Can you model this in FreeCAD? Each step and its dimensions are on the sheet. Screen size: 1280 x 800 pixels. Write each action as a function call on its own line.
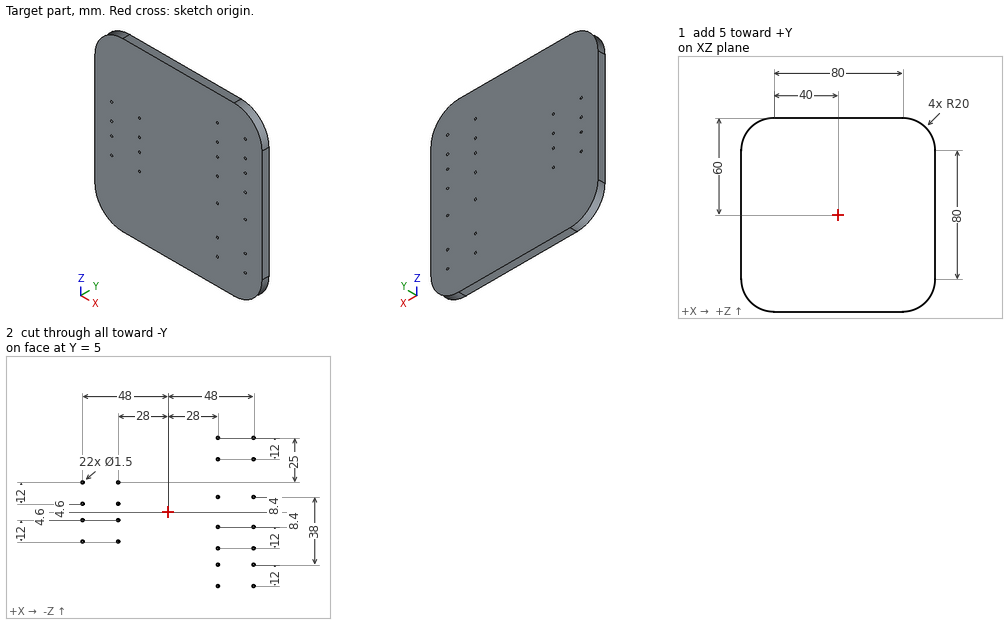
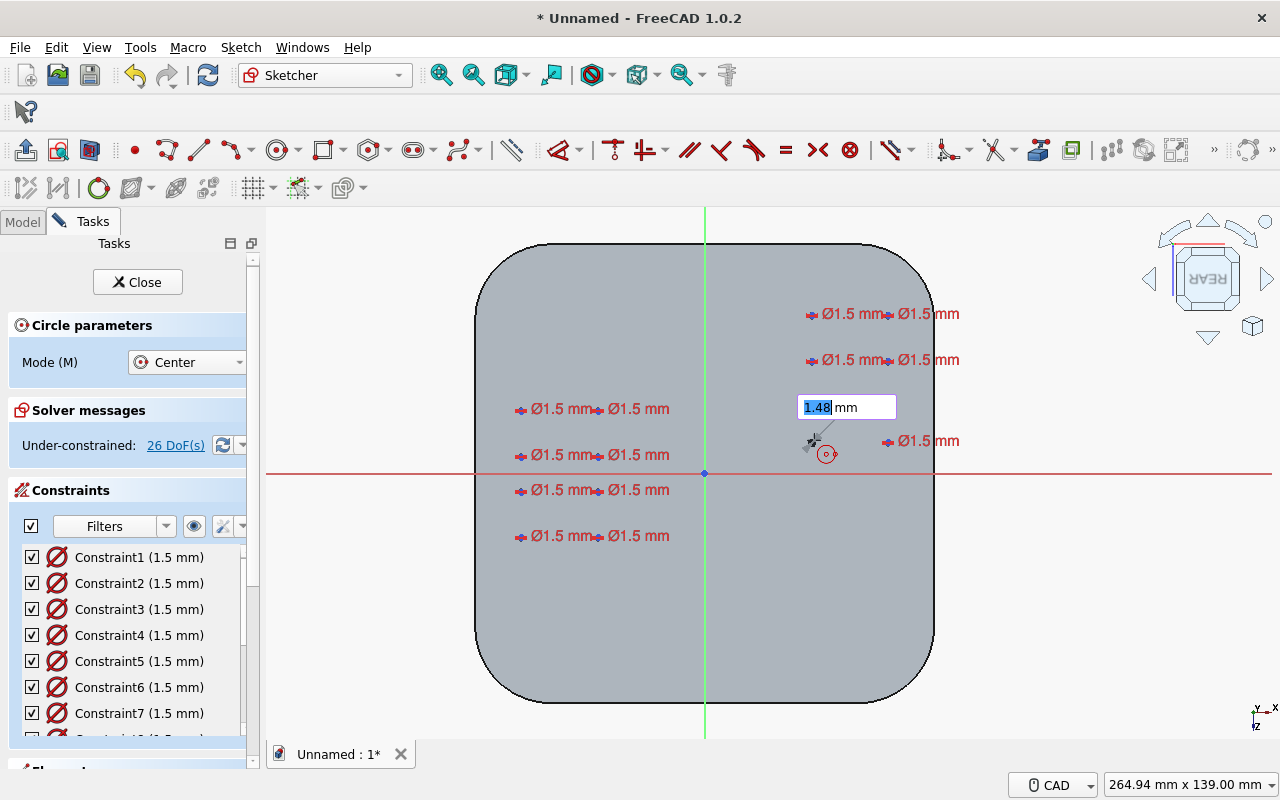
text(1.5)
key(Return)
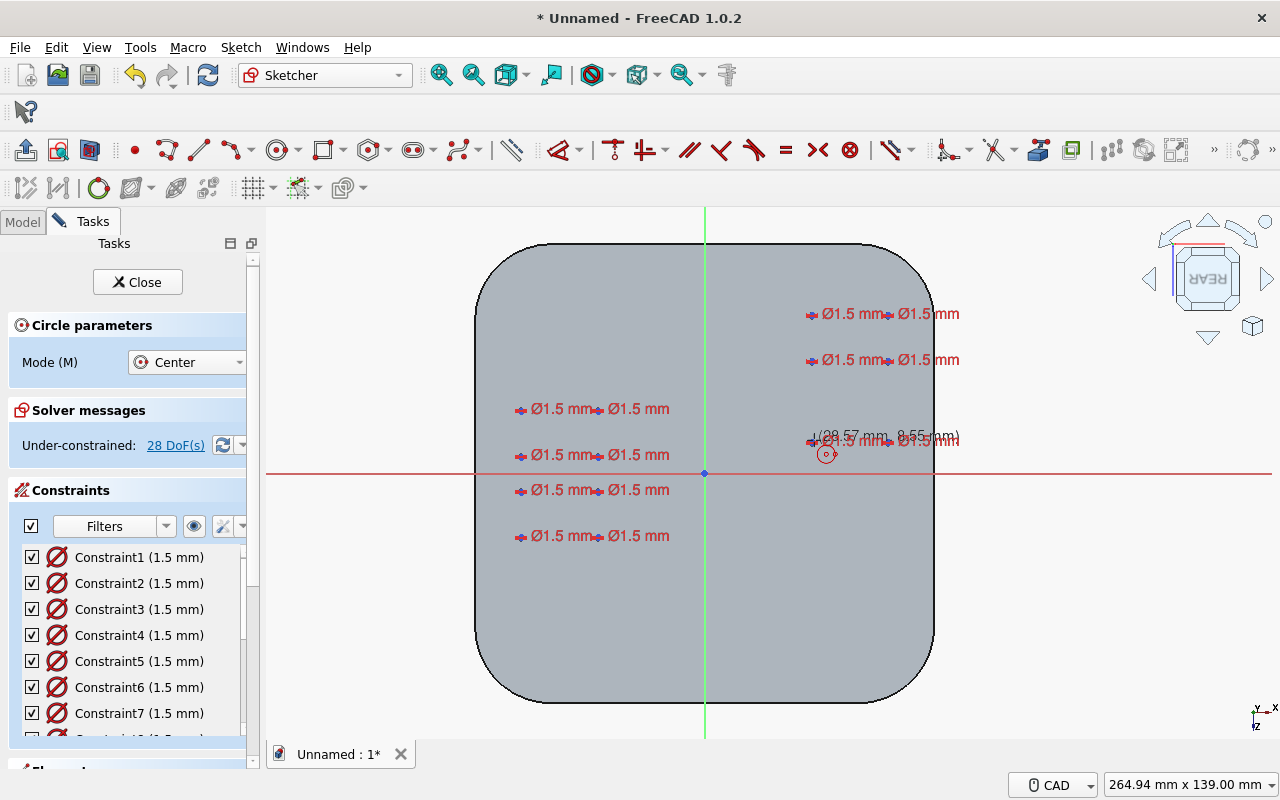
scroll(812, 506, up, 11)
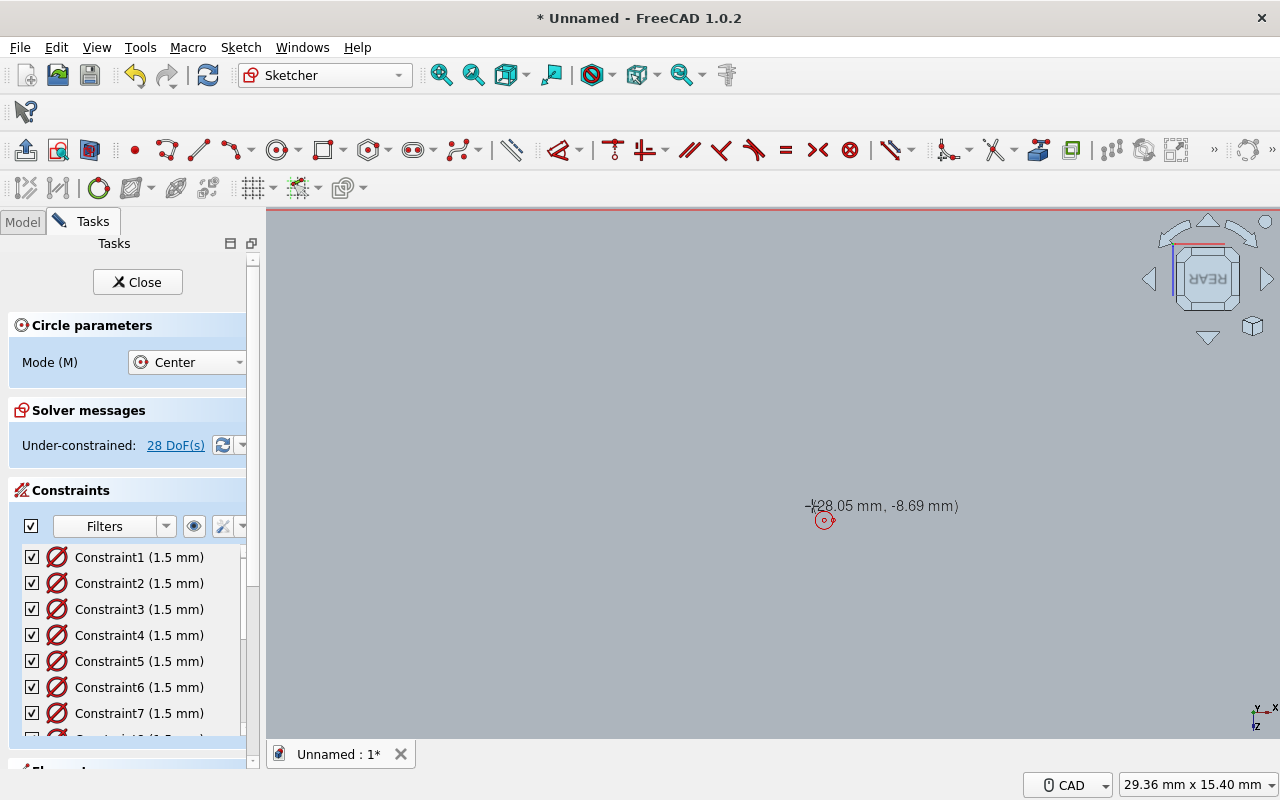
scroll(812, 506, down, 11)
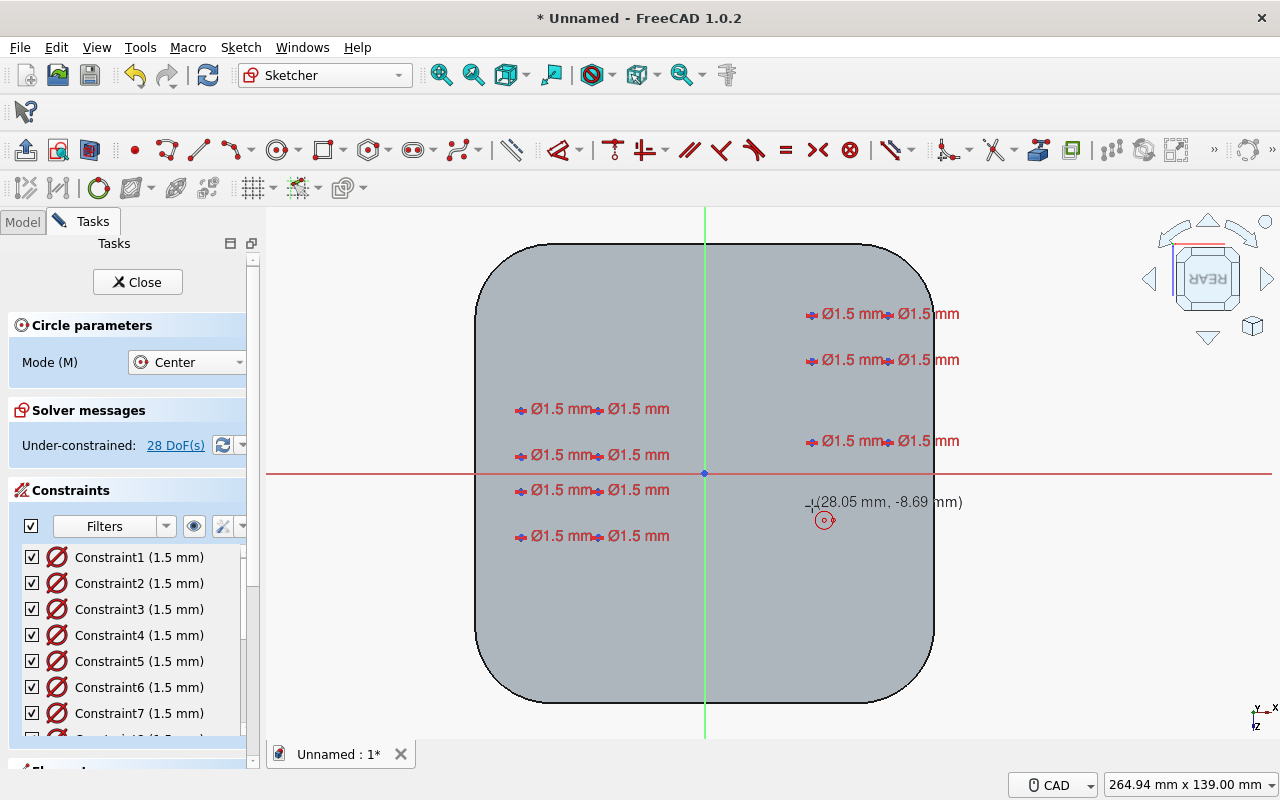
click(812, 506)
move(814, 504)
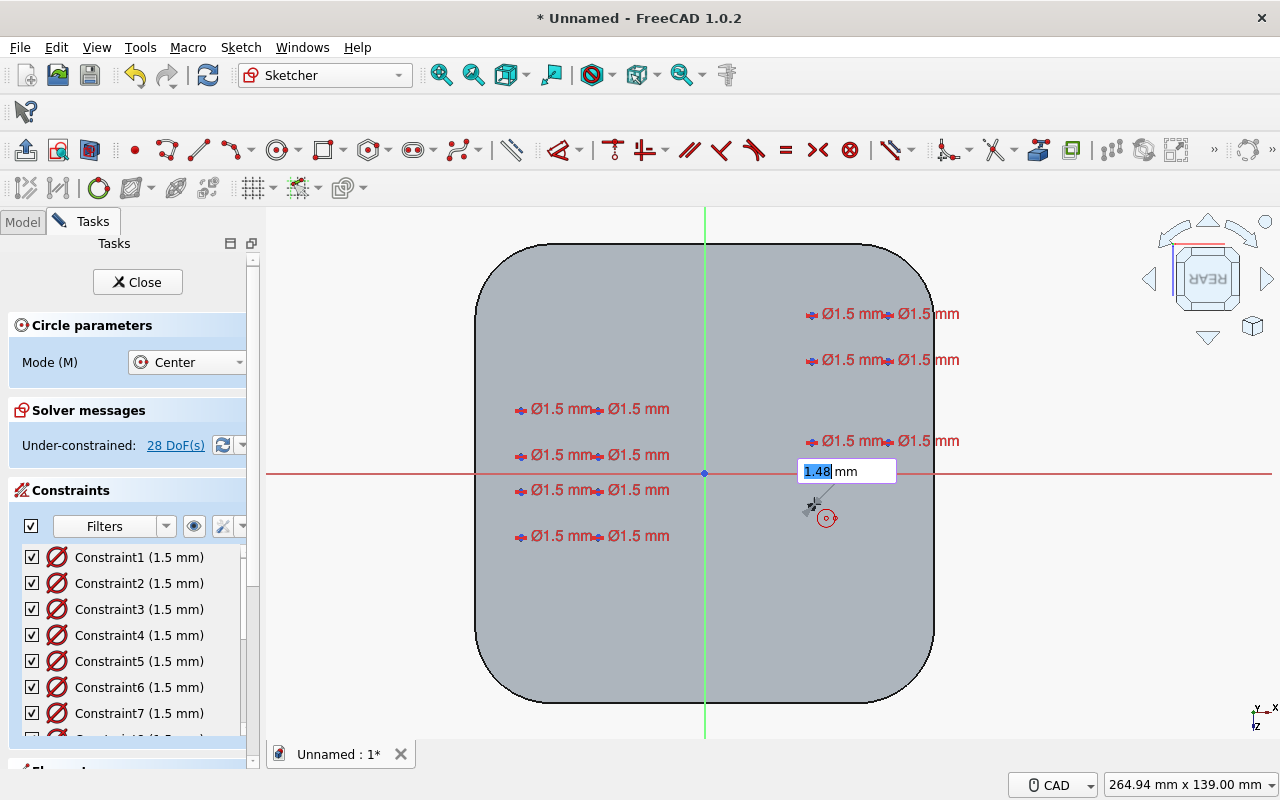
text(1.5)
key(Return)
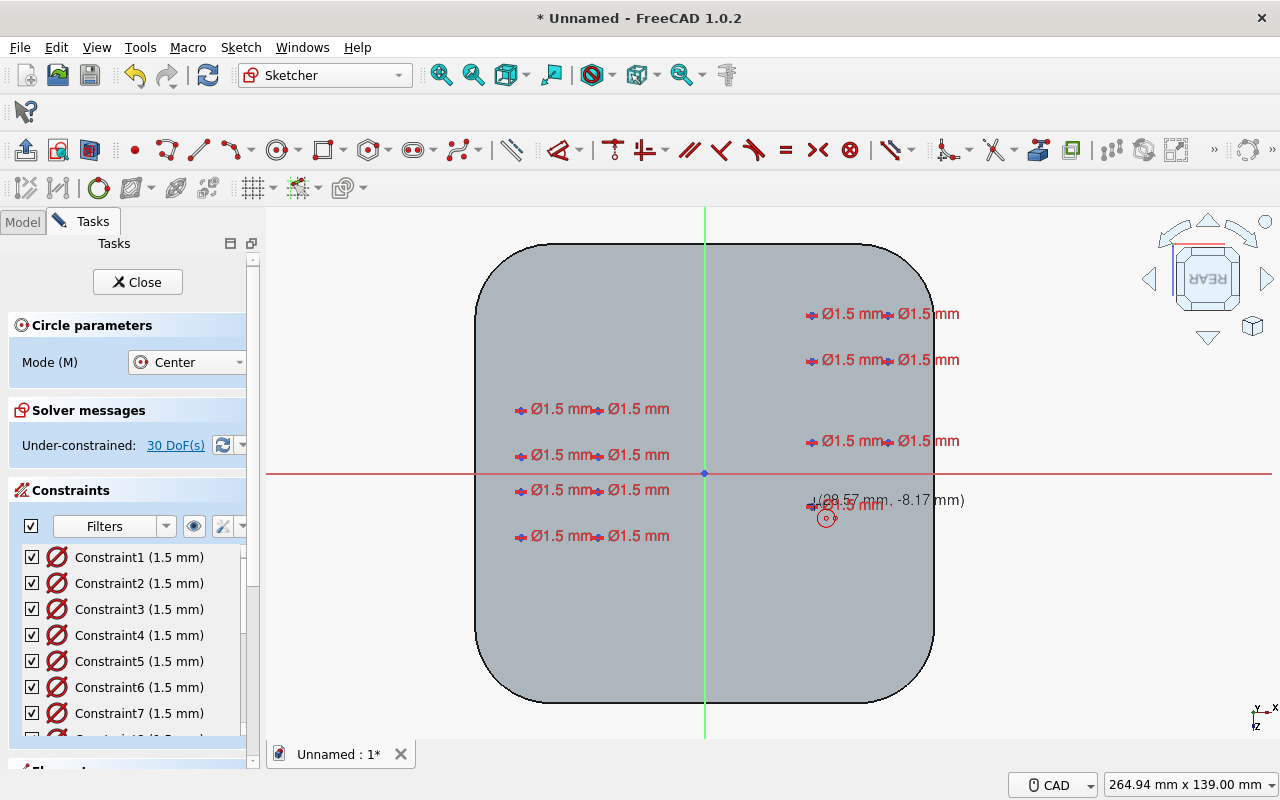
scroll(888, 506, up, 11)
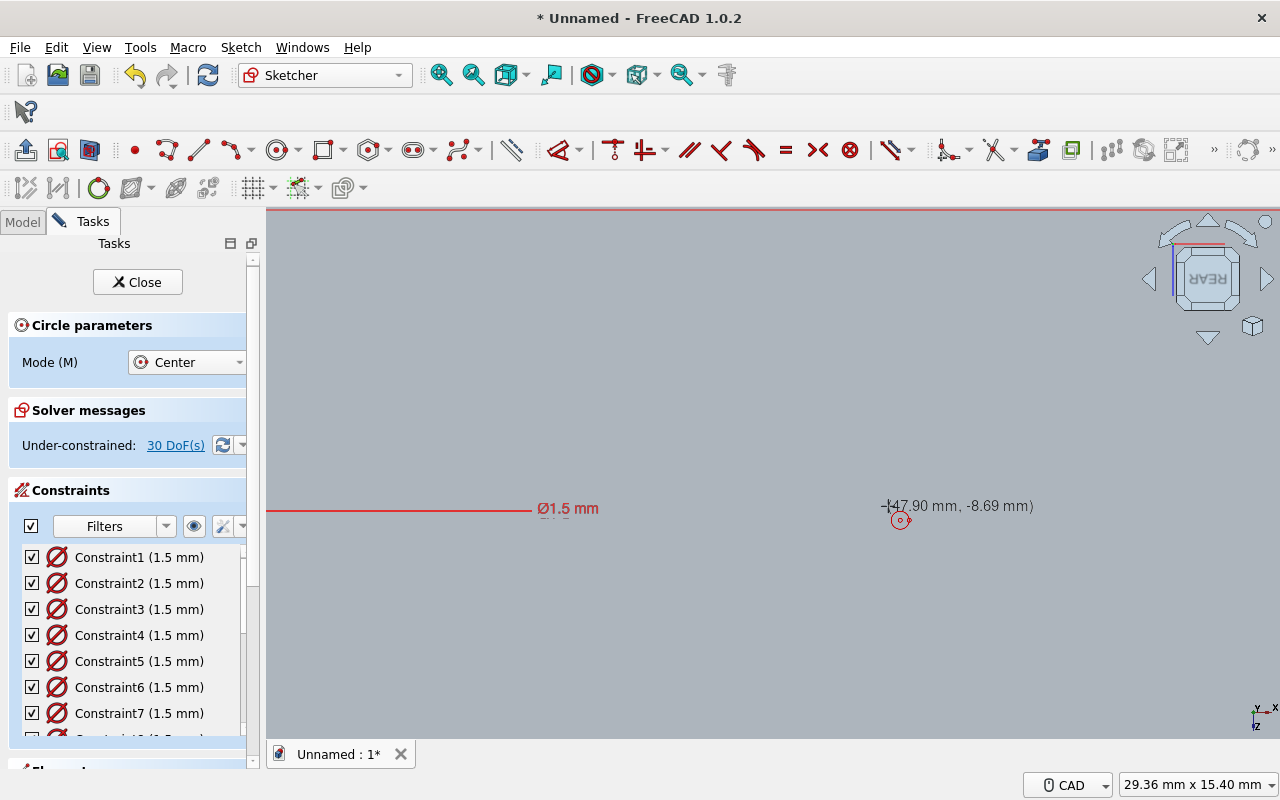
scroll(888, 506, down, 11)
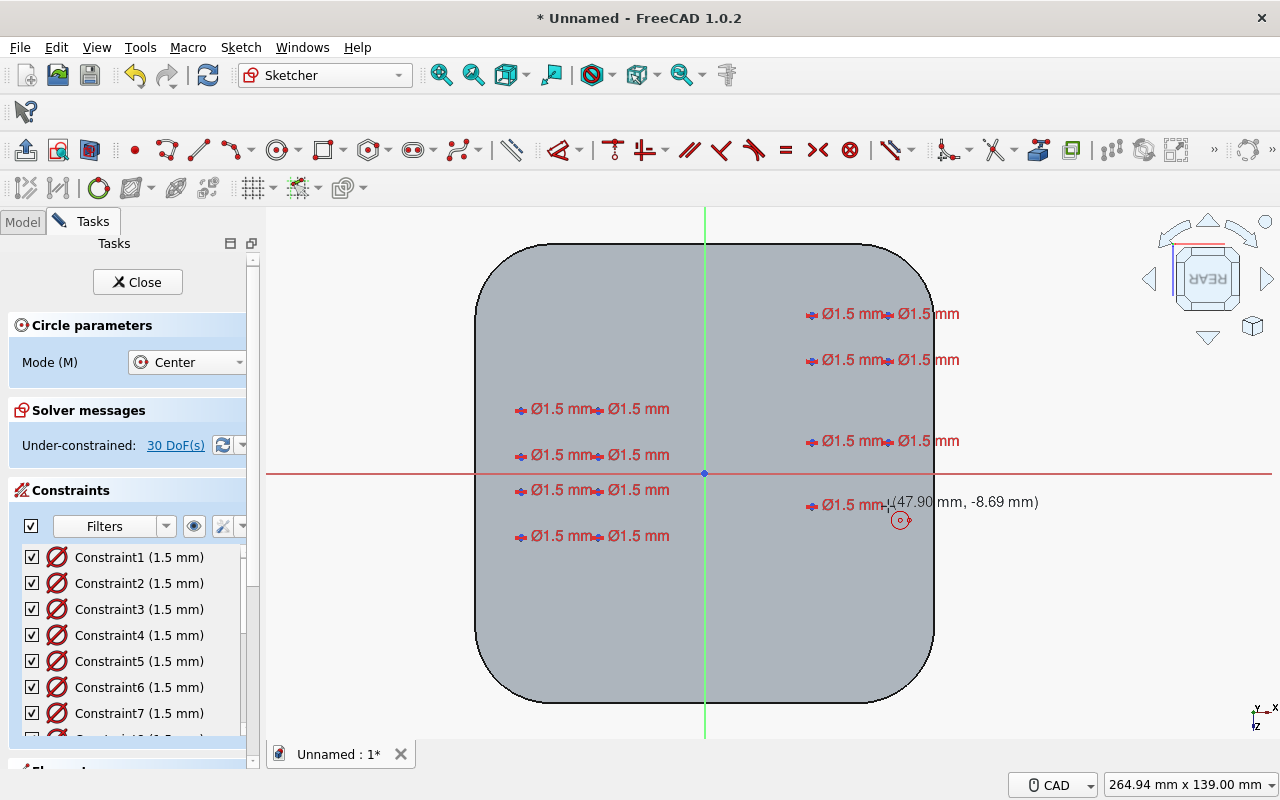
click(888, 506)
move(890, 504)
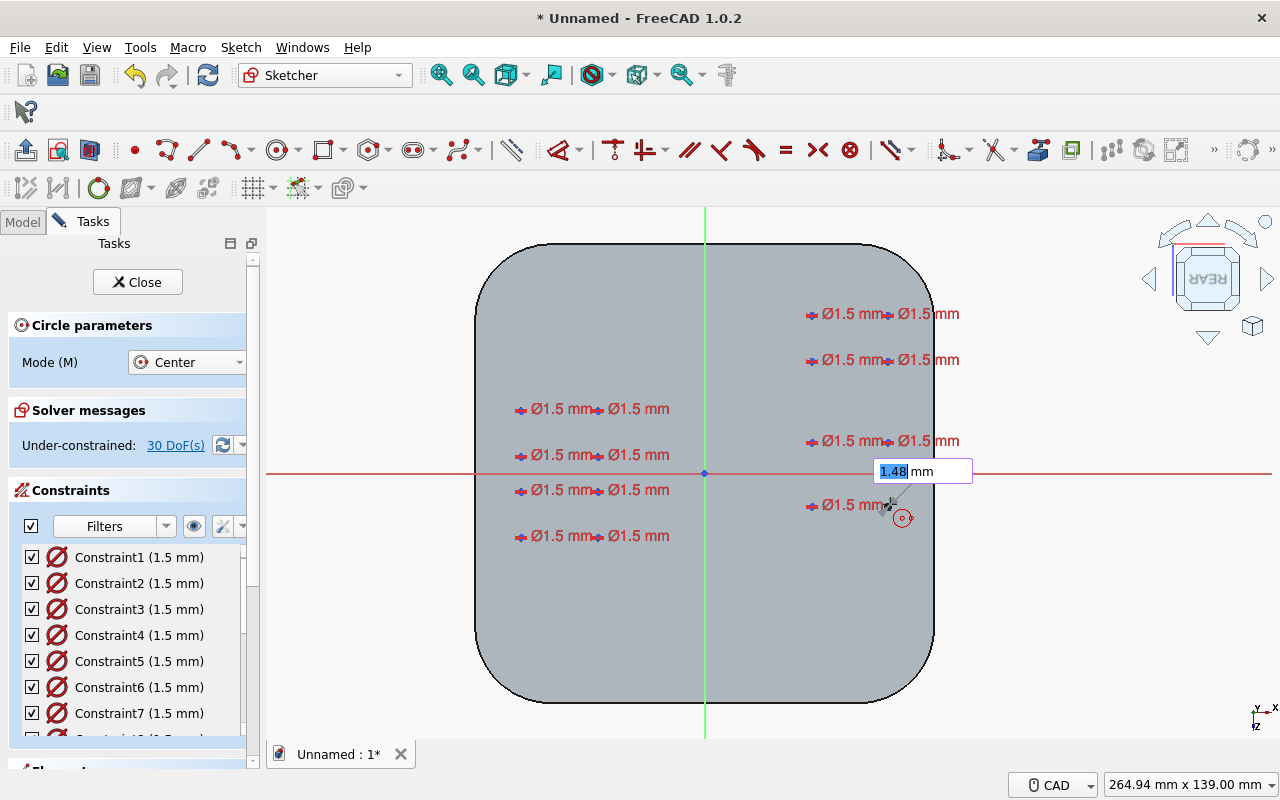
text(1.5)
key(Return)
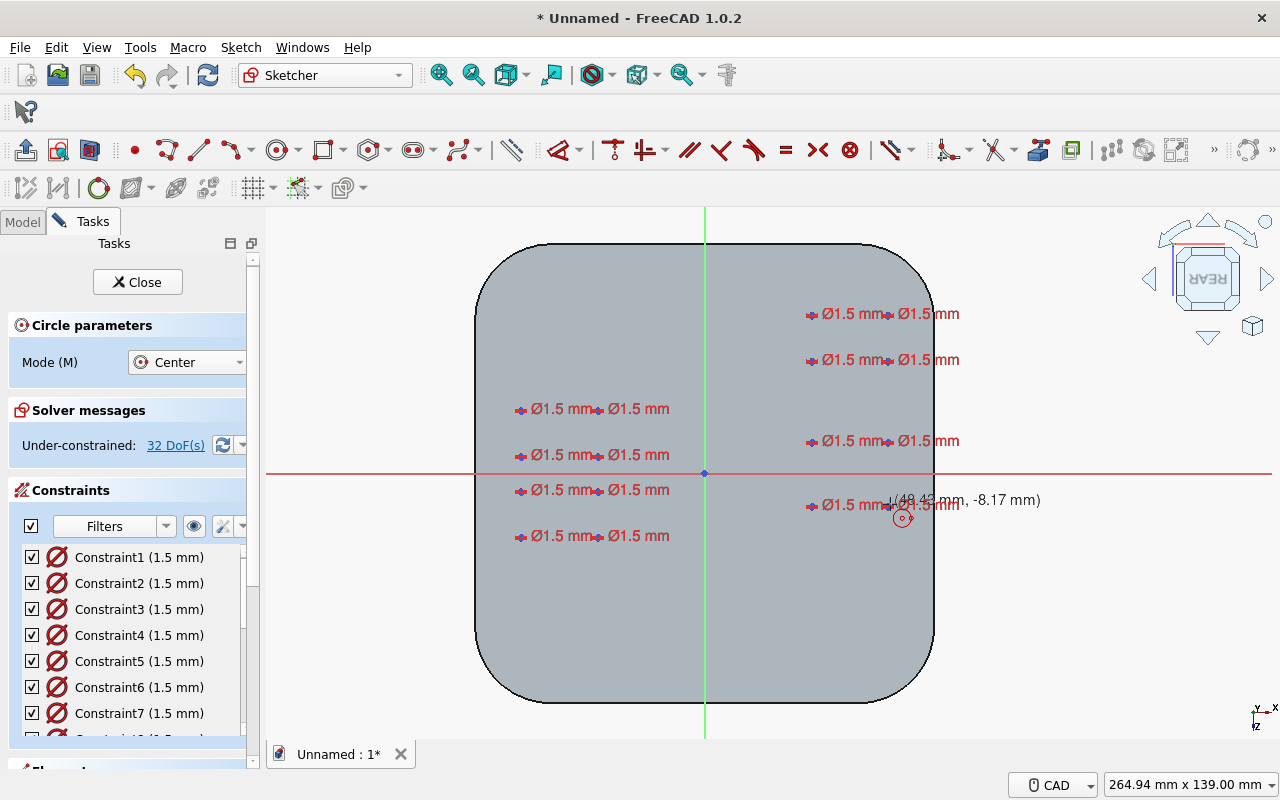
scroll(812, 552, up, 11)